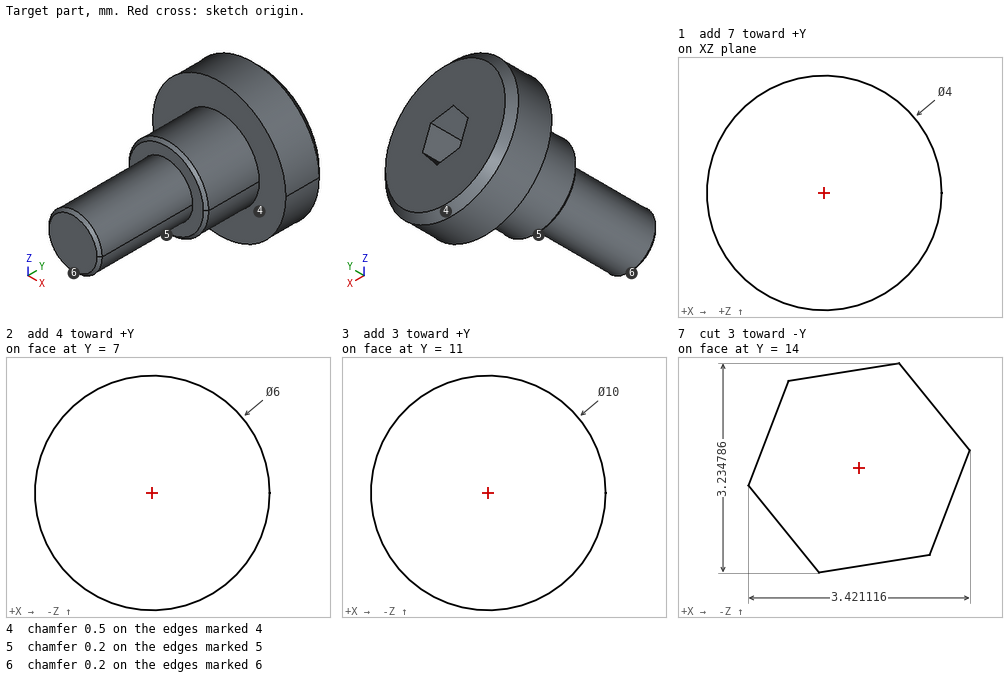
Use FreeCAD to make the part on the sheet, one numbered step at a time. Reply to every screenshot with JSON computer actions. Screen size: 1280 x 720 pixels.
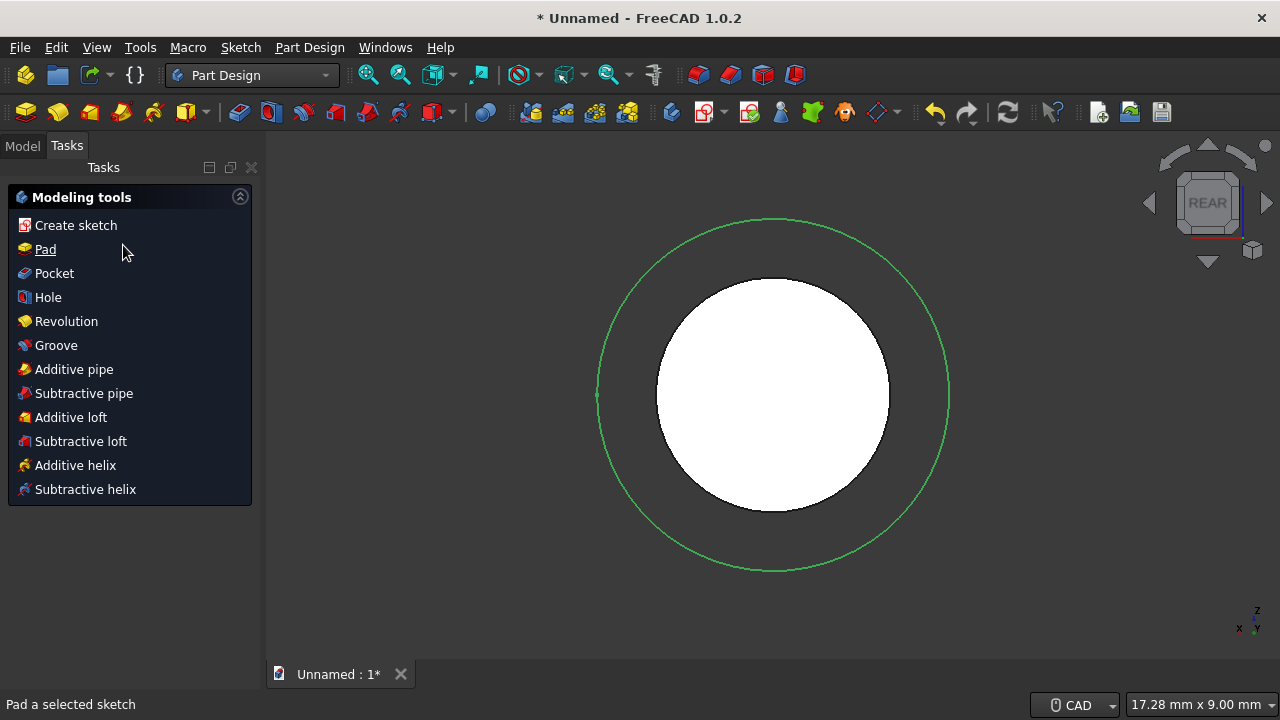
{"action": "left_click", "coordinate": [26, 112]}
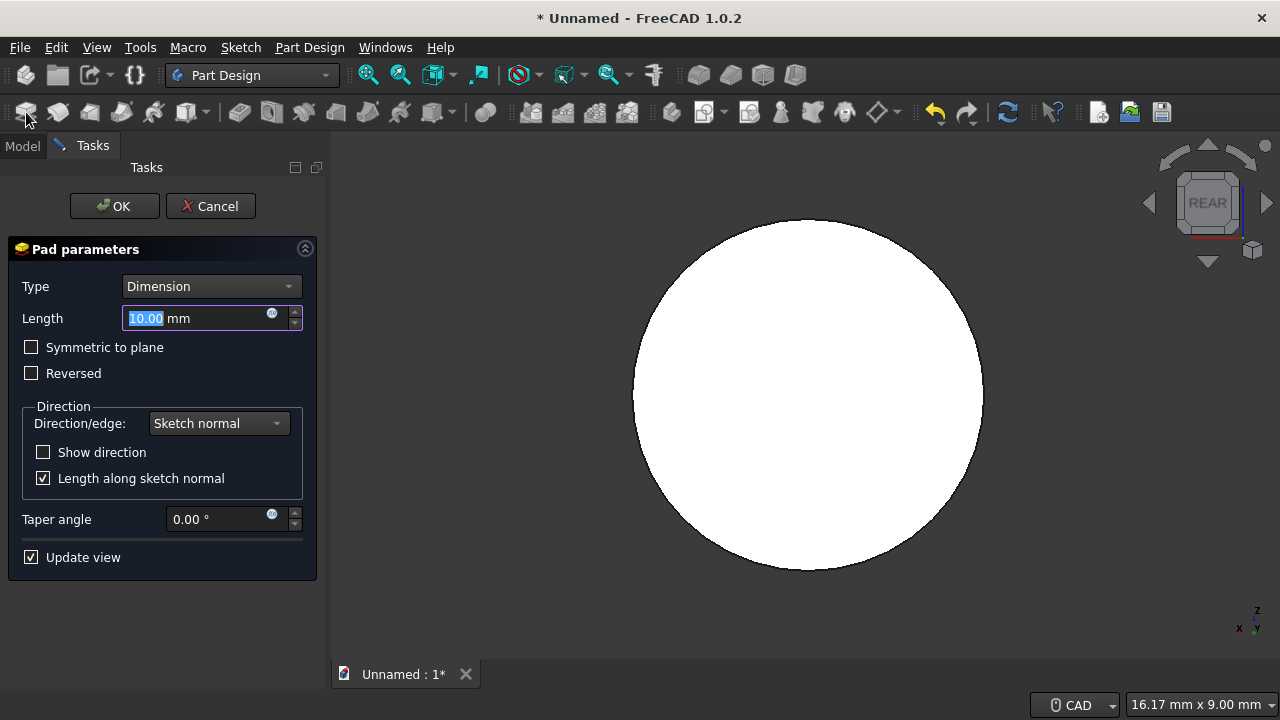
{"action": "type", "text": "4"}
{"action": "key", "text": "Tab"}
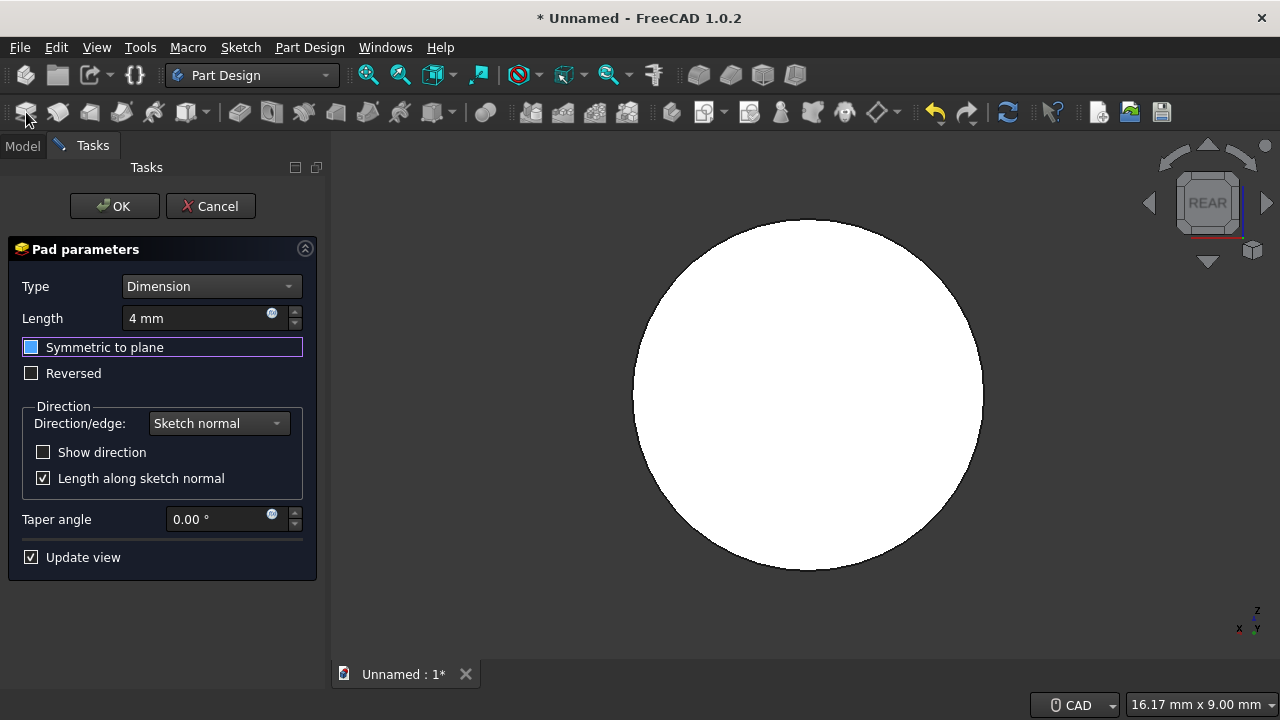
{"action": "left_click", "coordinate": [115, 206]}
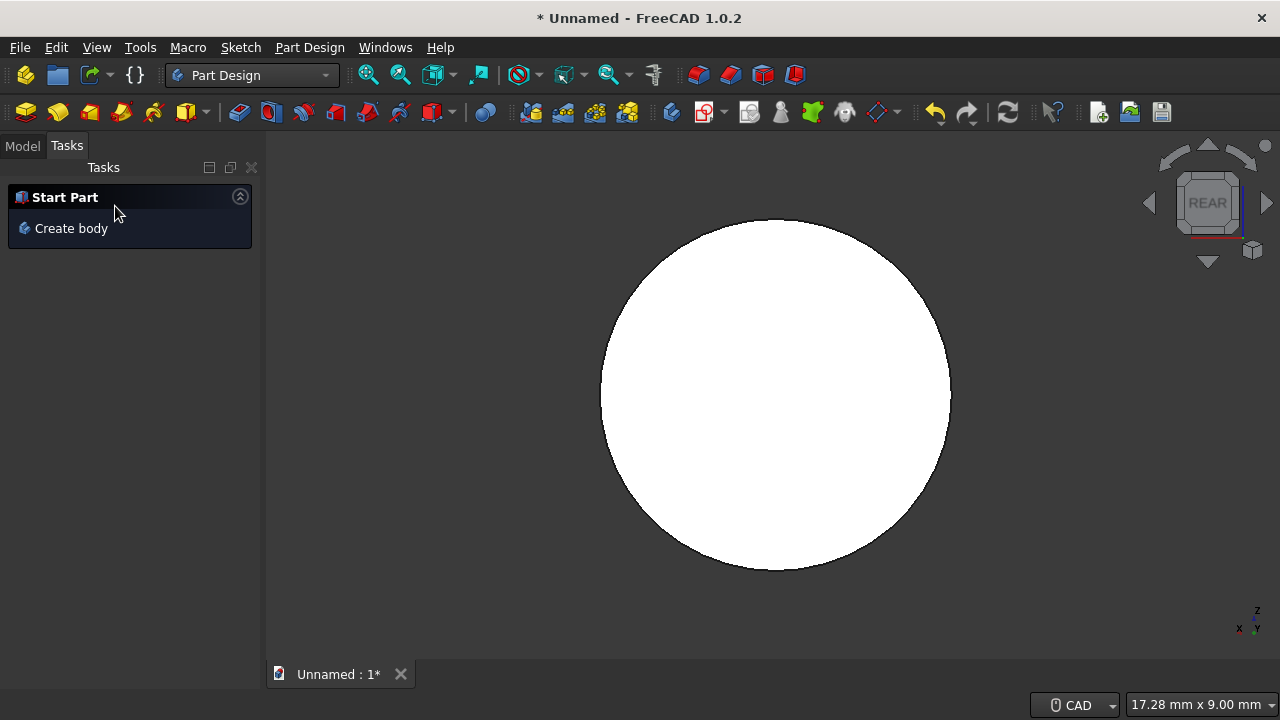
{"action": "left_click", "coordinate": [776, 394]}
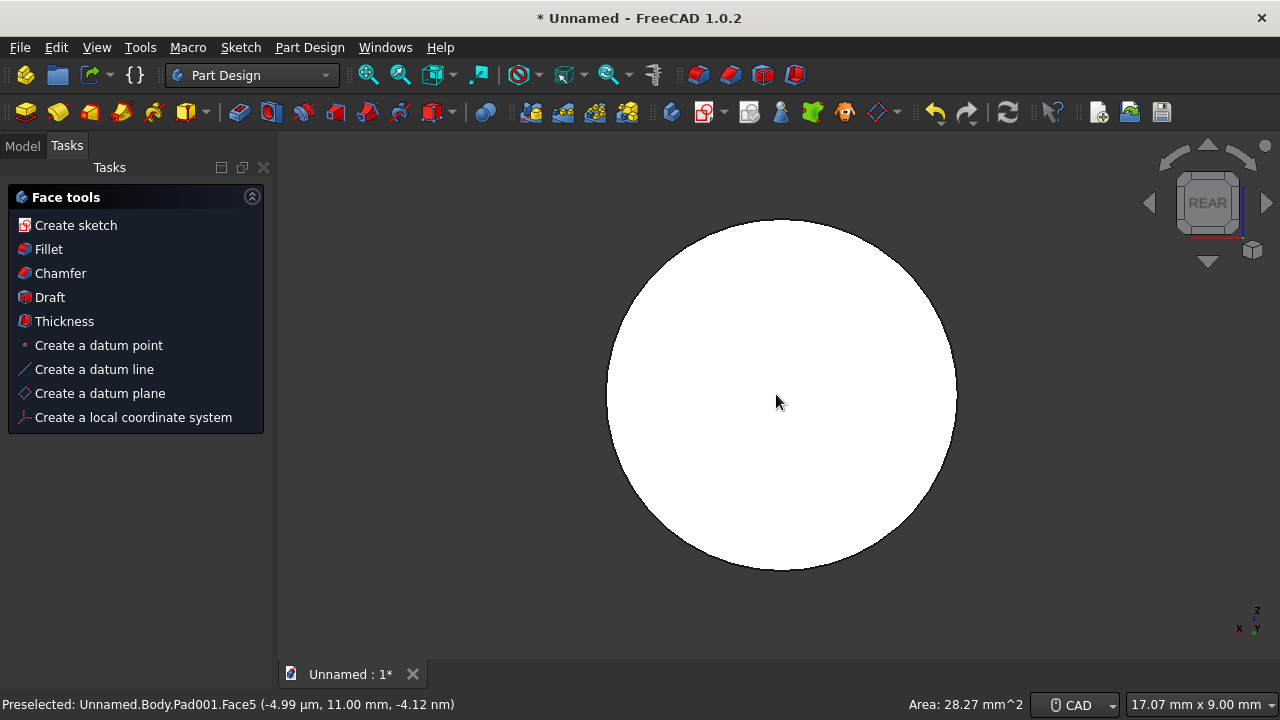
{"action": "left_click", "coordinate": [704, 112]}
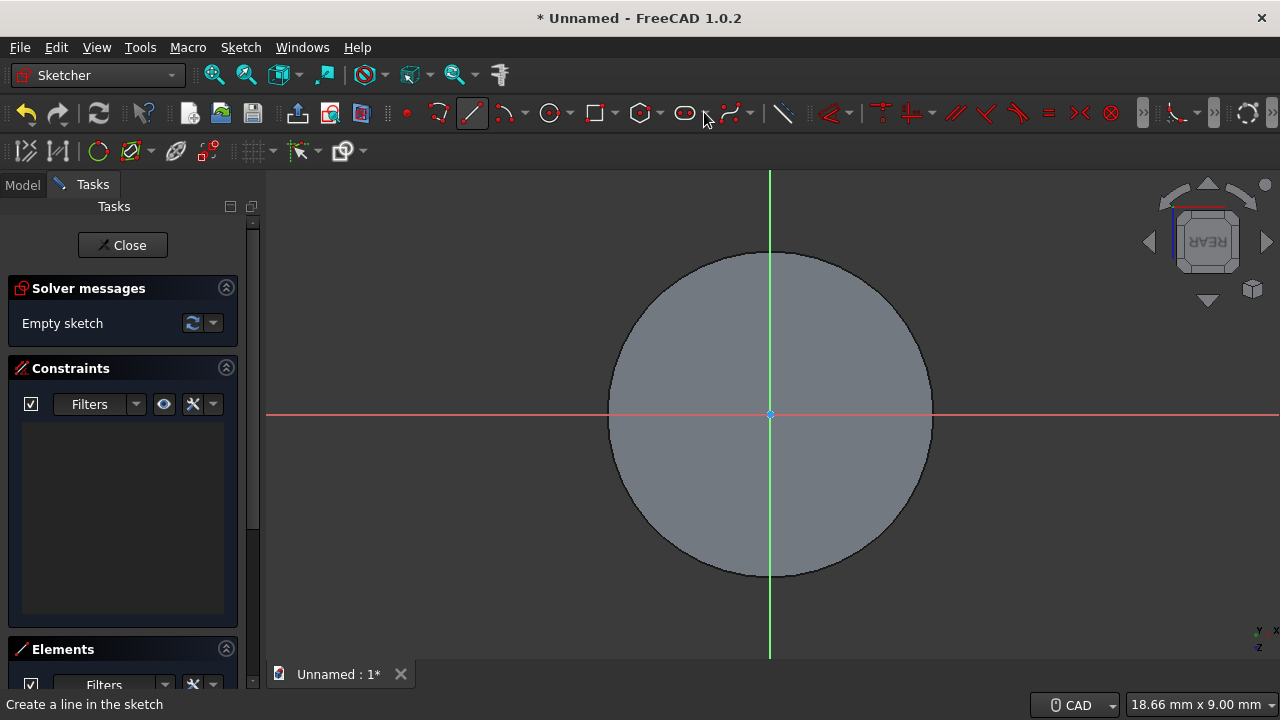
{"action": "scroll", "coordinate": [624, 414], "scroll_direction": "down", "scroll_amount": 3}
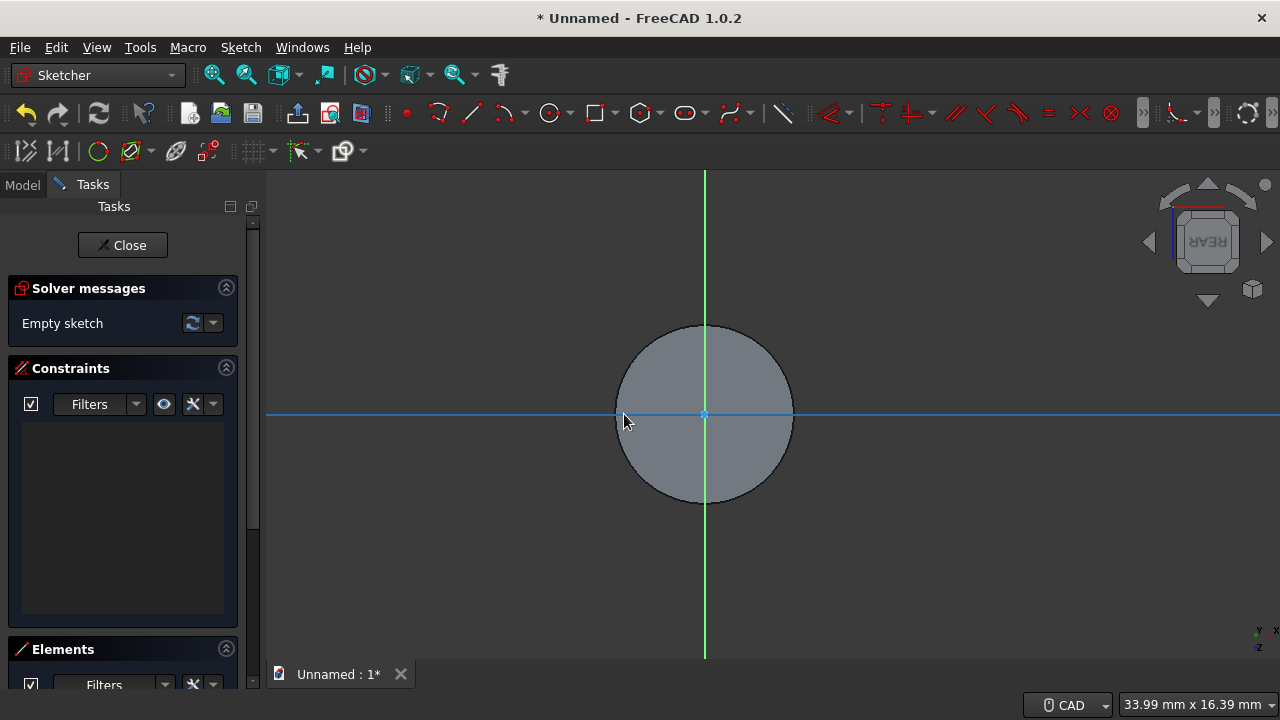
{"action": "key", "text": "g c"}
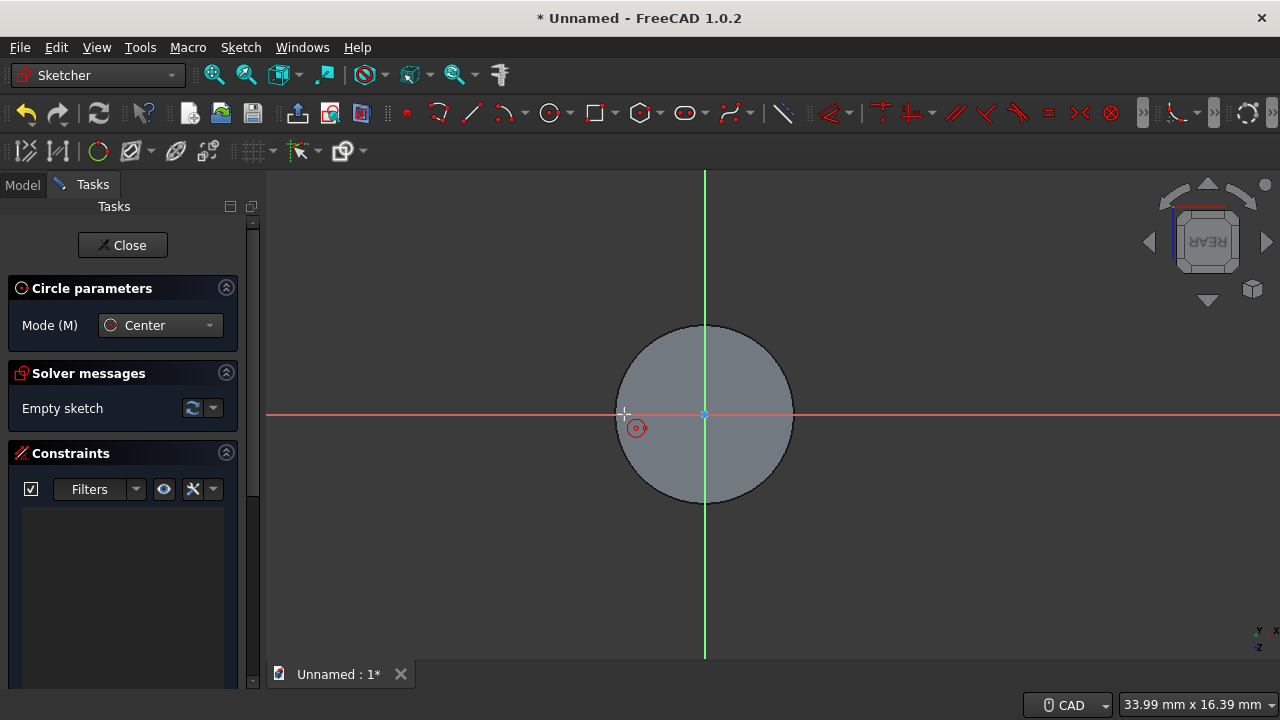
{"action": "left_click", "coordinate": [705, 415]}
{"action": "mouse_move", "coordinate": [810, 309]}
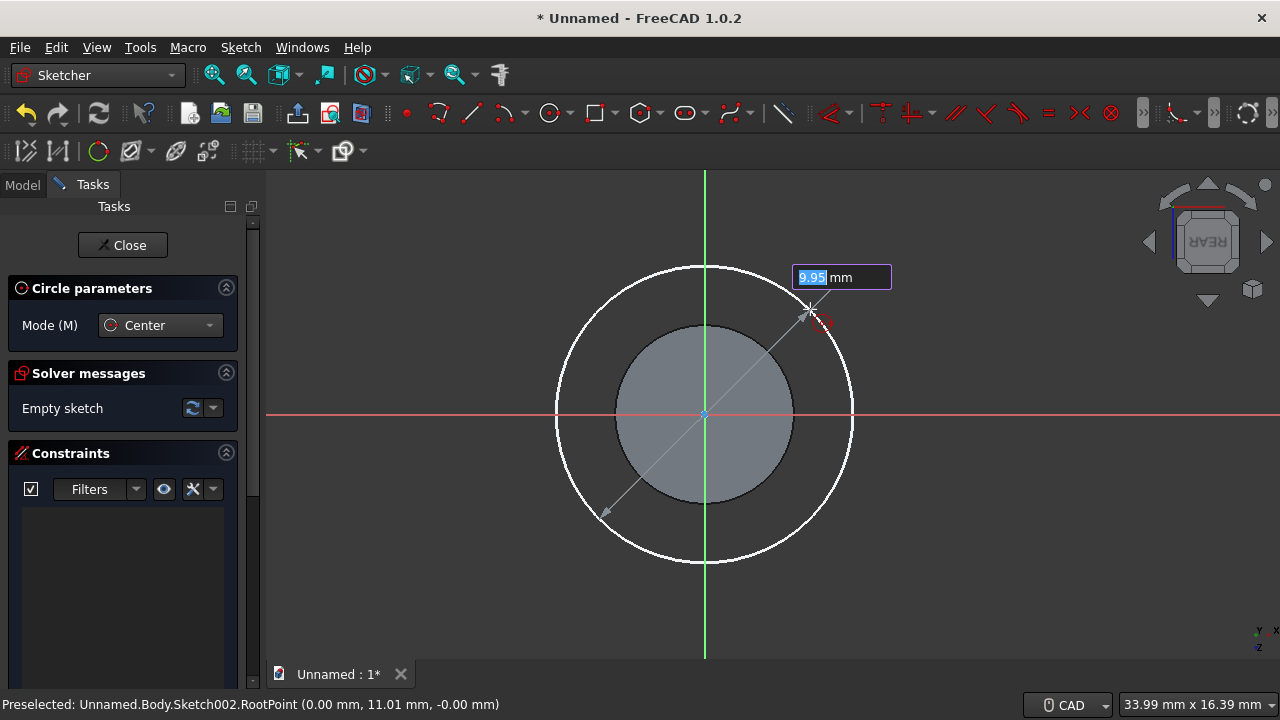
{"action": "type", "text": "10"}
{"action": "key", "text": "Return"}
{"action": "key", "text": "Escape"}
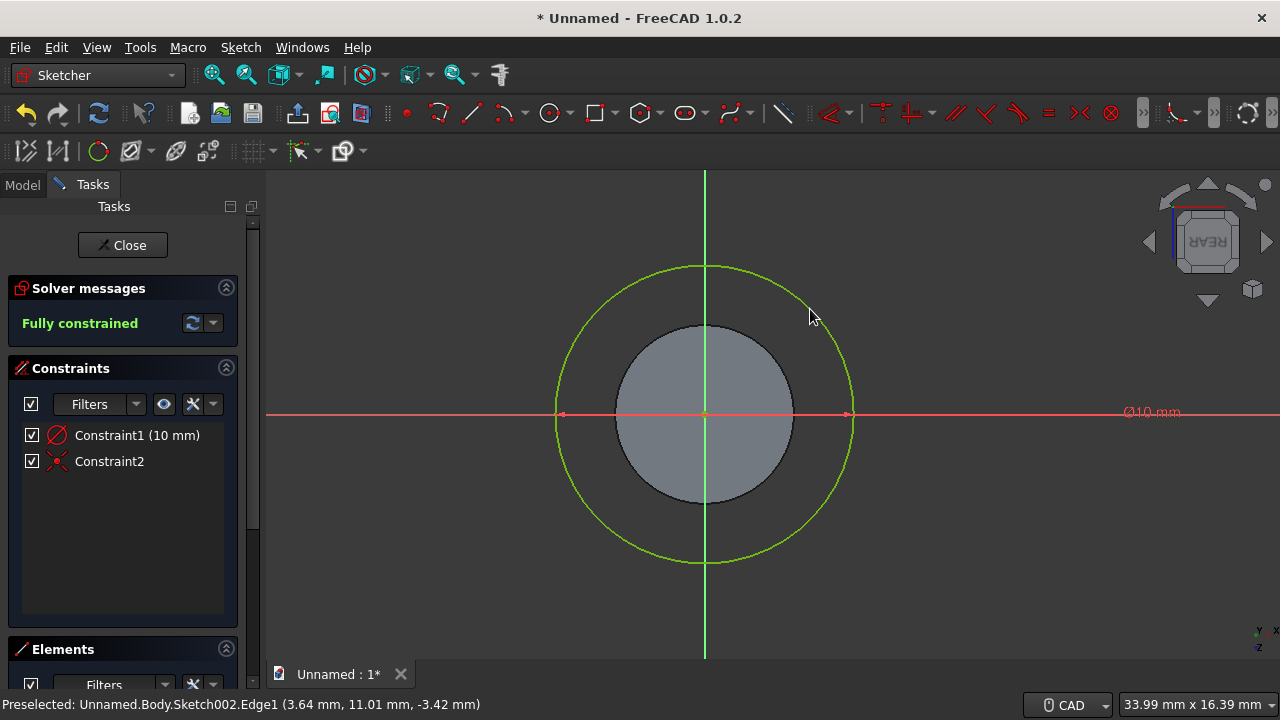
{"action": "left_click", "coordinate": [123, 245]}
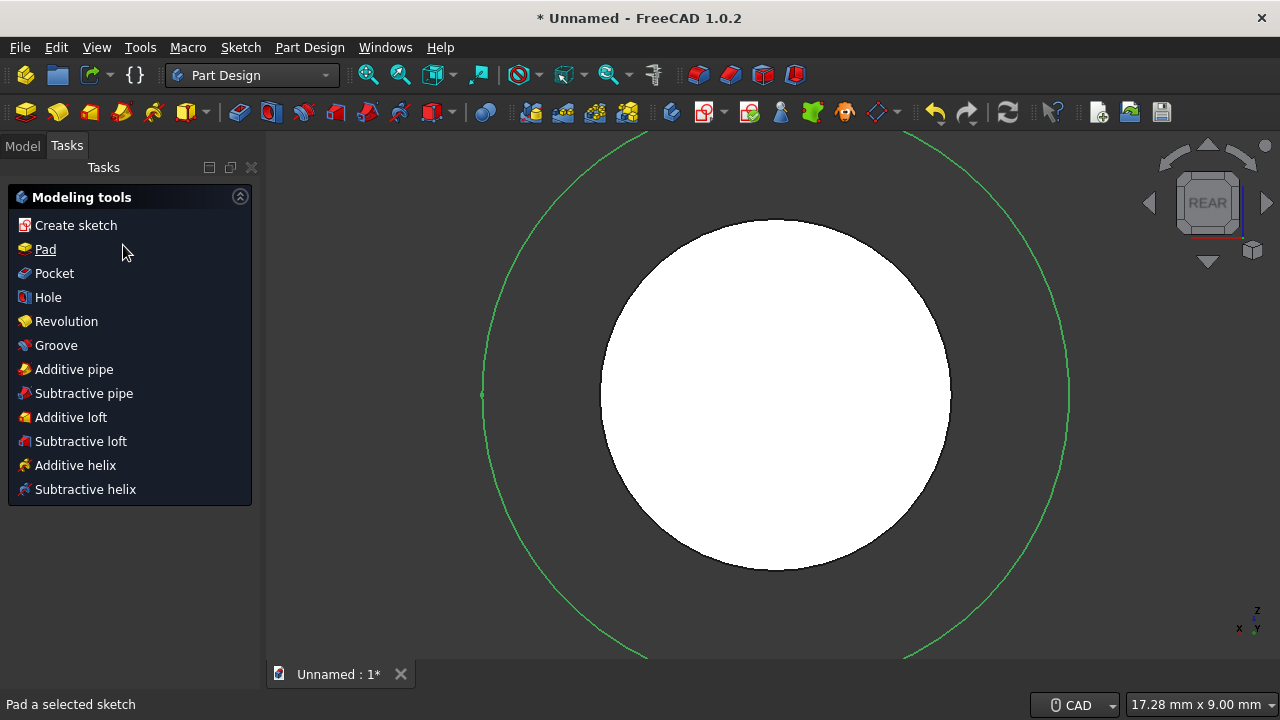
{"action": "left_click", "coordinate": [26, 112]}